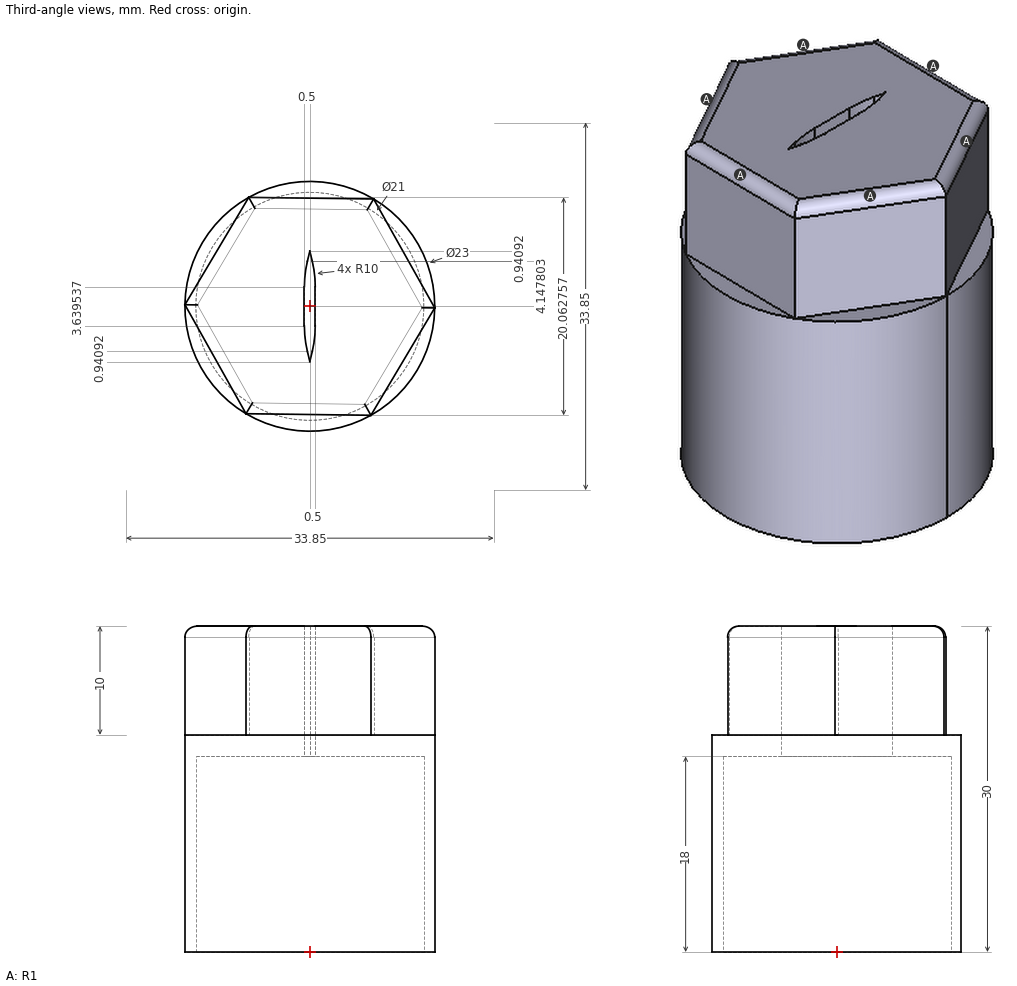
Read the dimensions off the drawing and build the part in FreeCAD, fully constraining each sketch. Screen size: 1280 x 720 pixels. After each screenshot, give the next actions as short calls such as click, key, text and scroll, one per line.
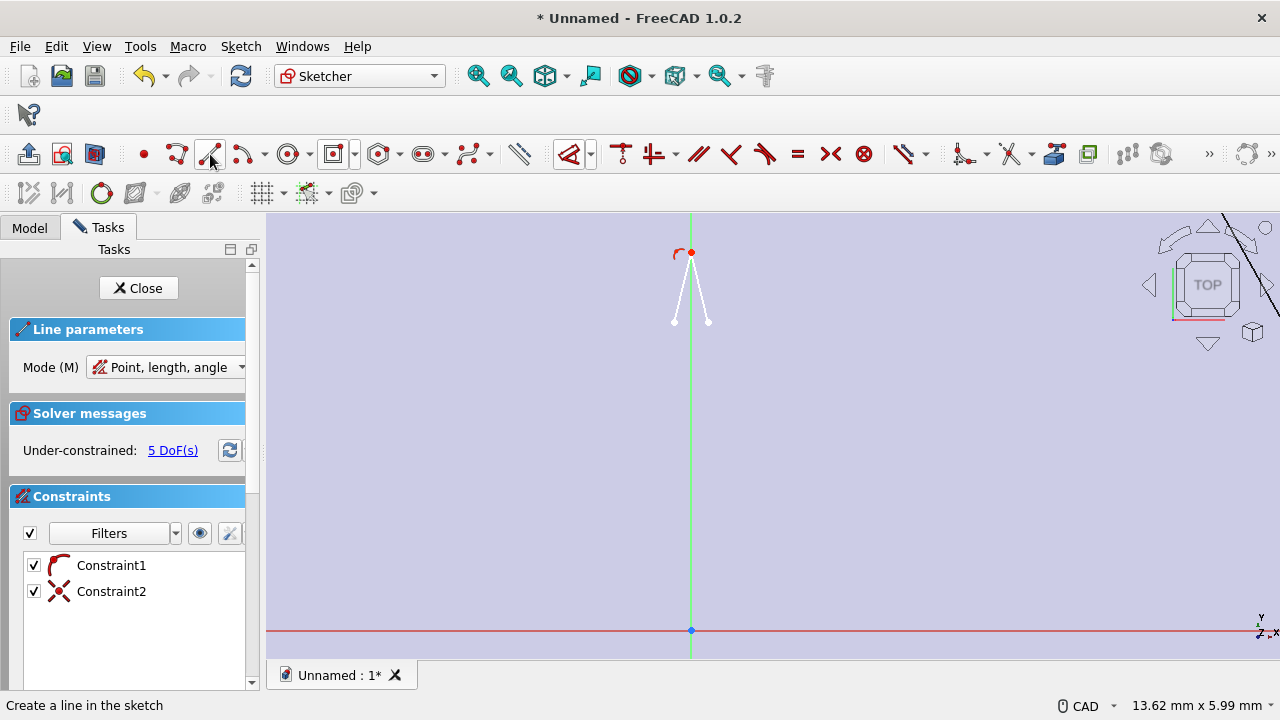
click(654, 495)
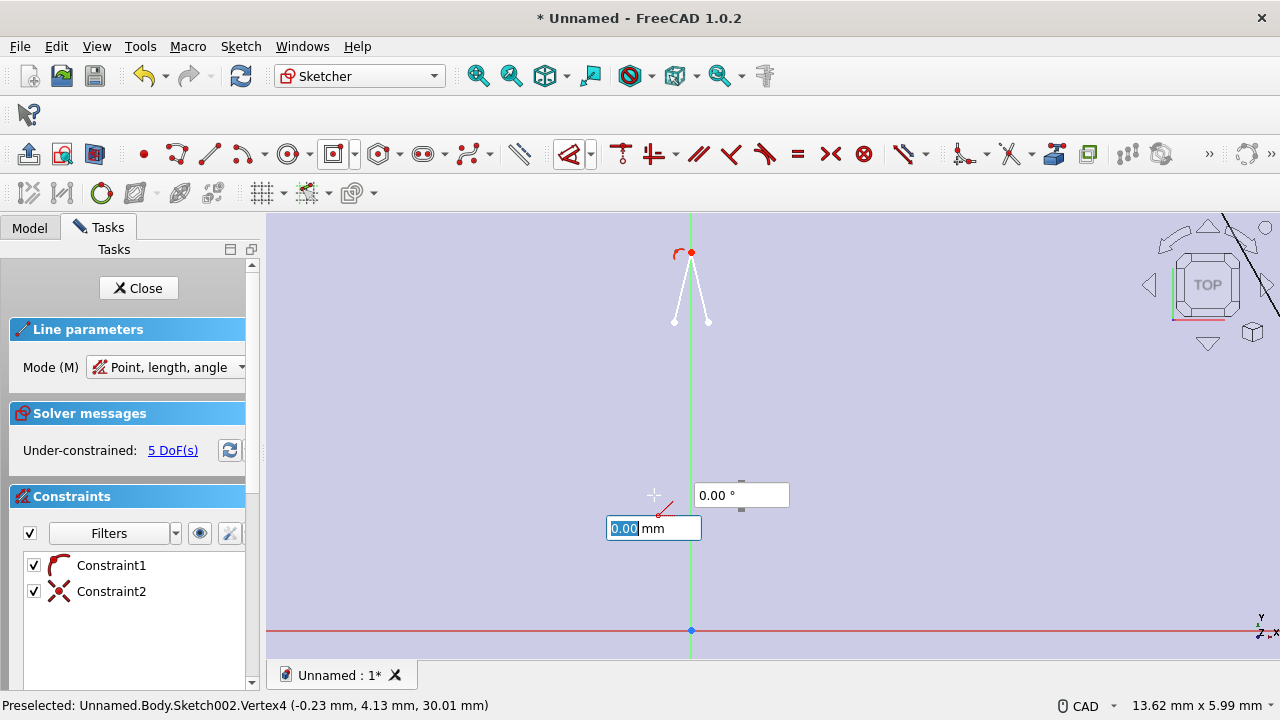
scroll(712, 323, down, 5)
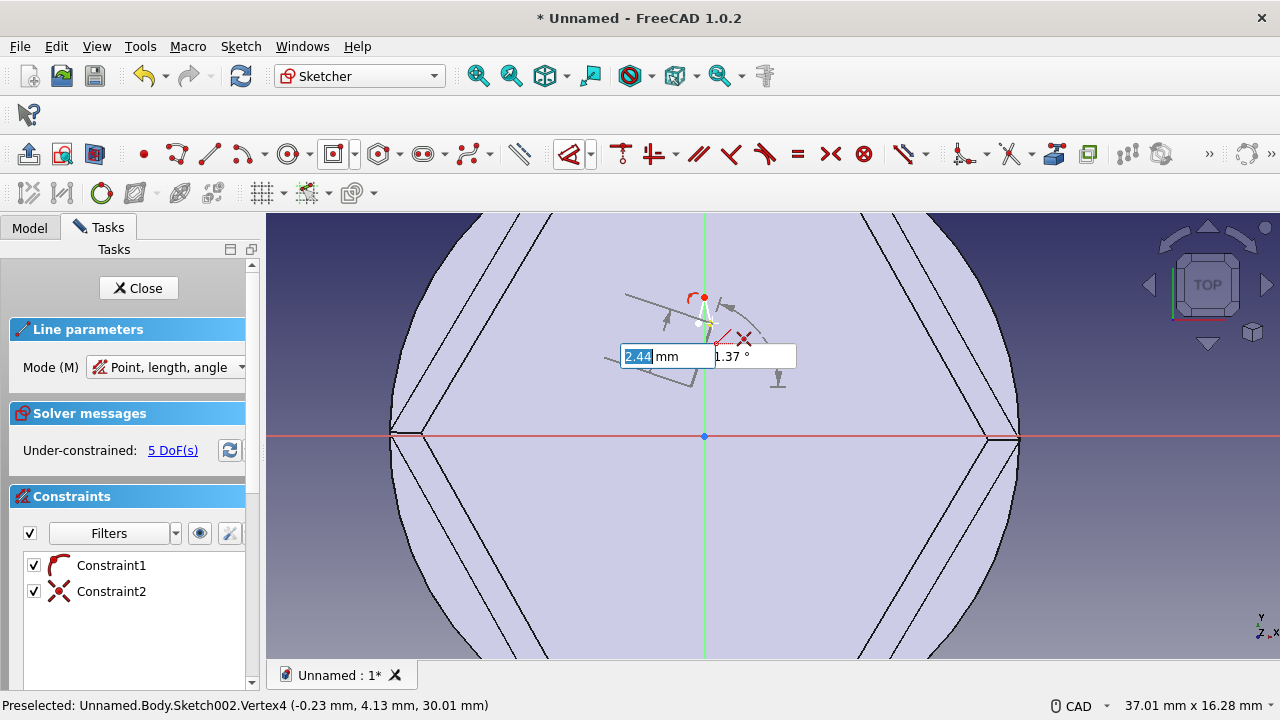
click(691, 486)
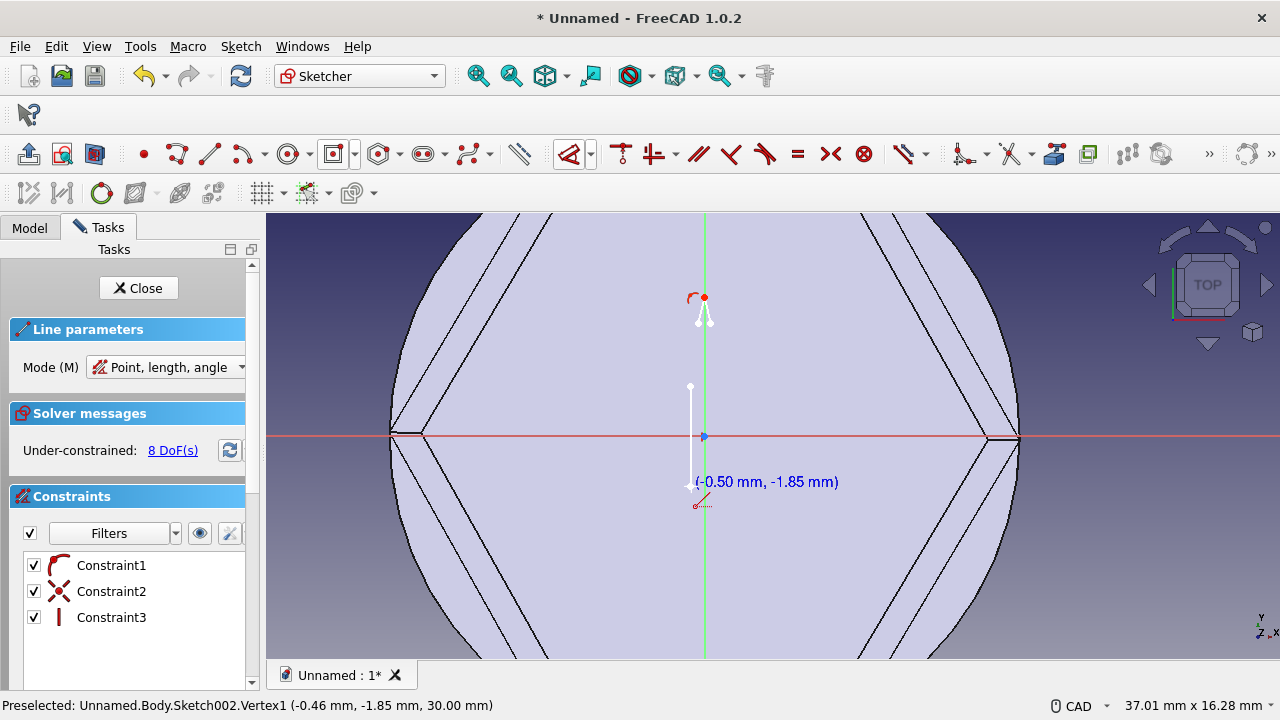
click(177, 154)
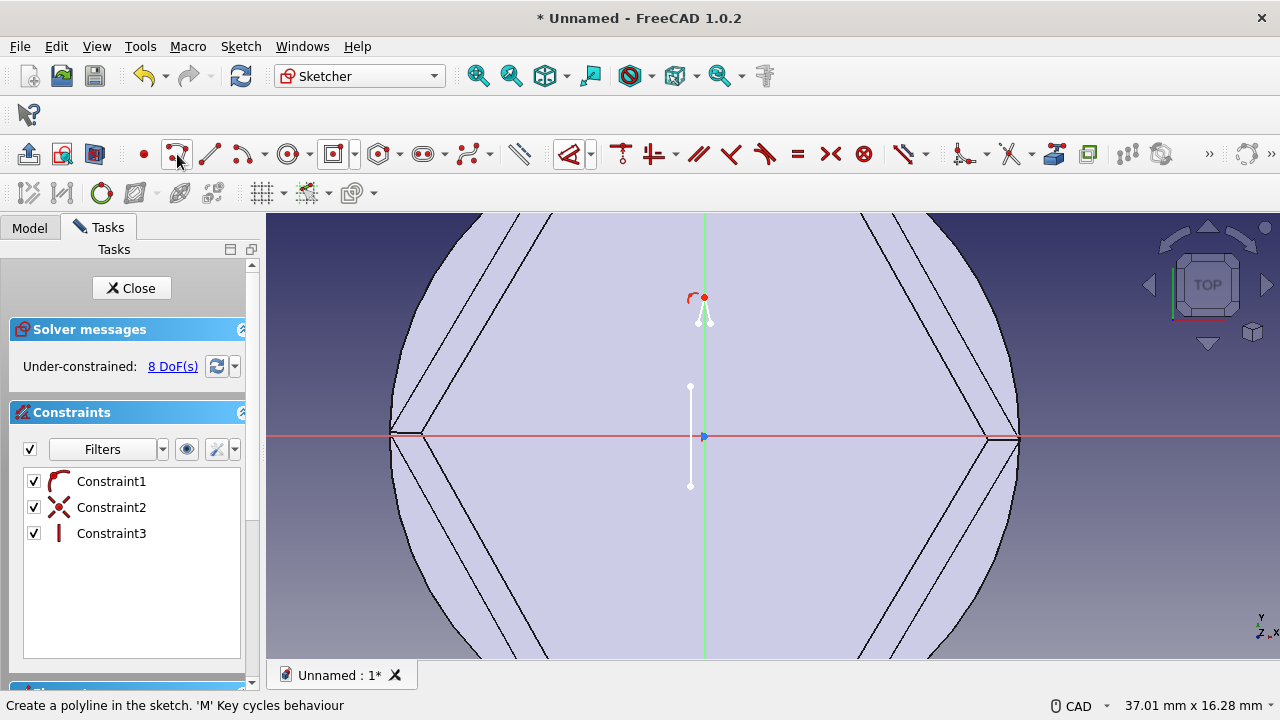
scroll(698, 550, up, 5)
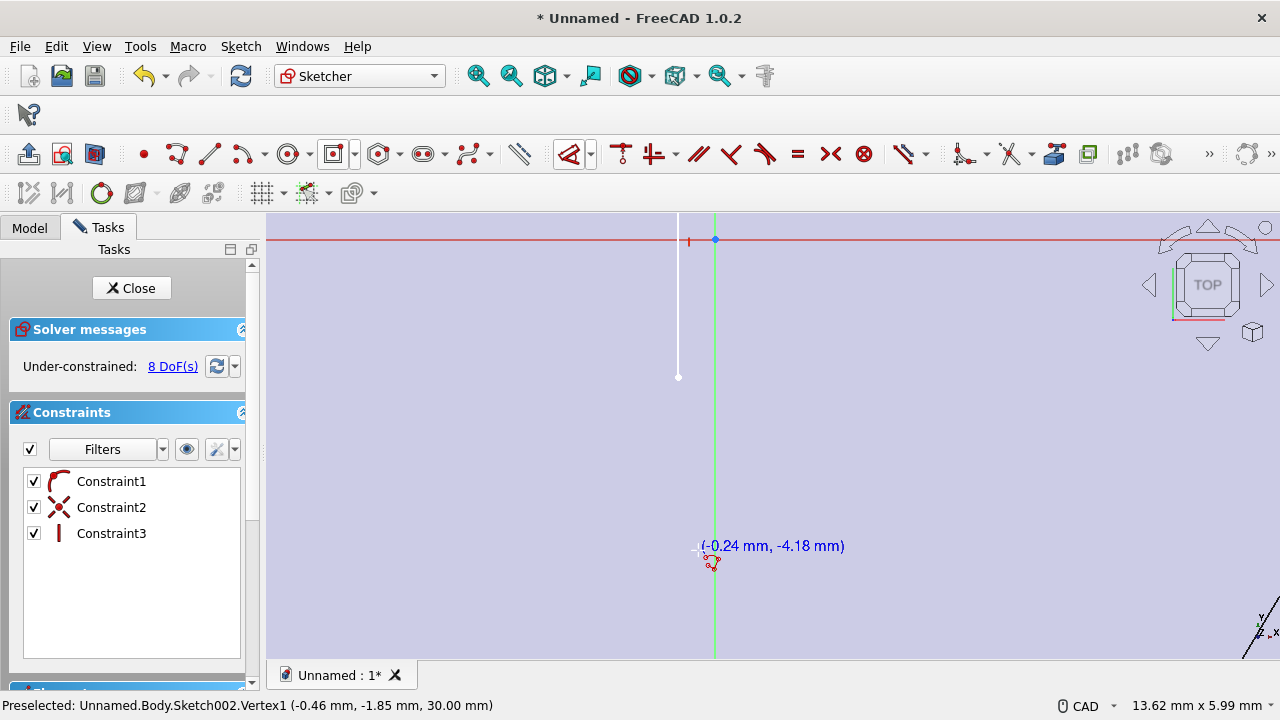
click(698, 549)
click(715, 619)
click(732, 549)
right_click(732, 549)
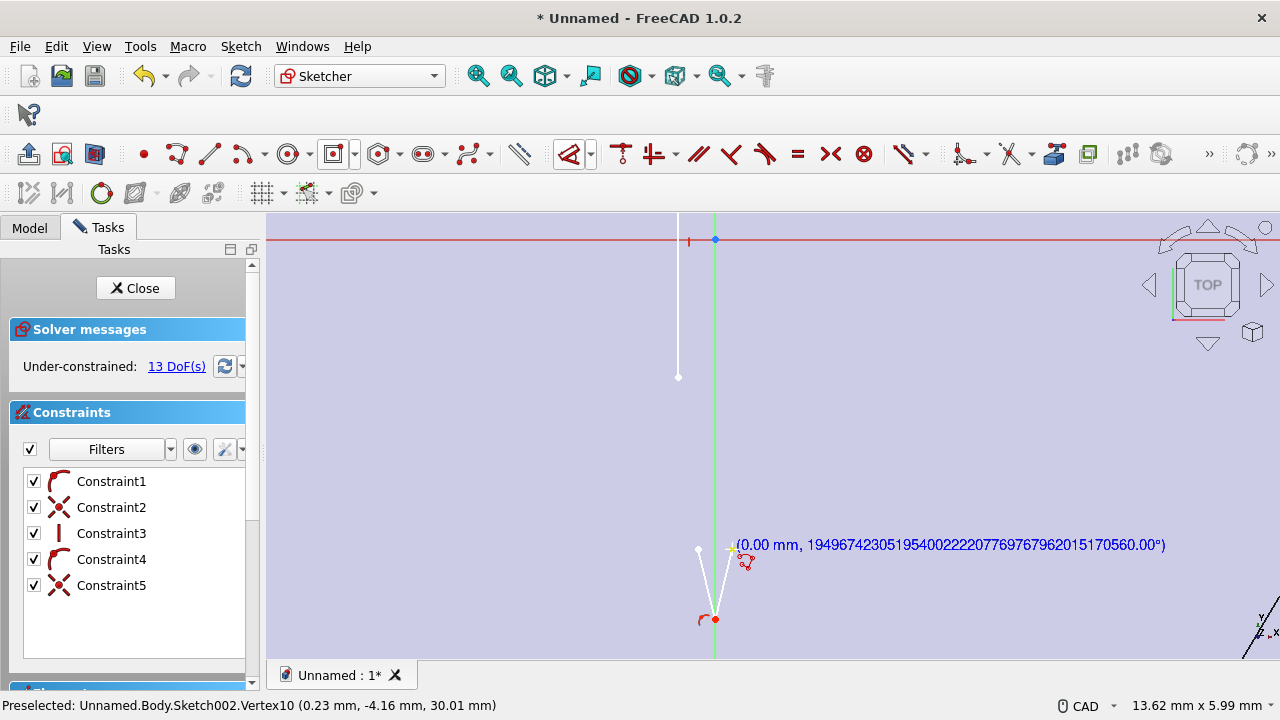
click(210, 154)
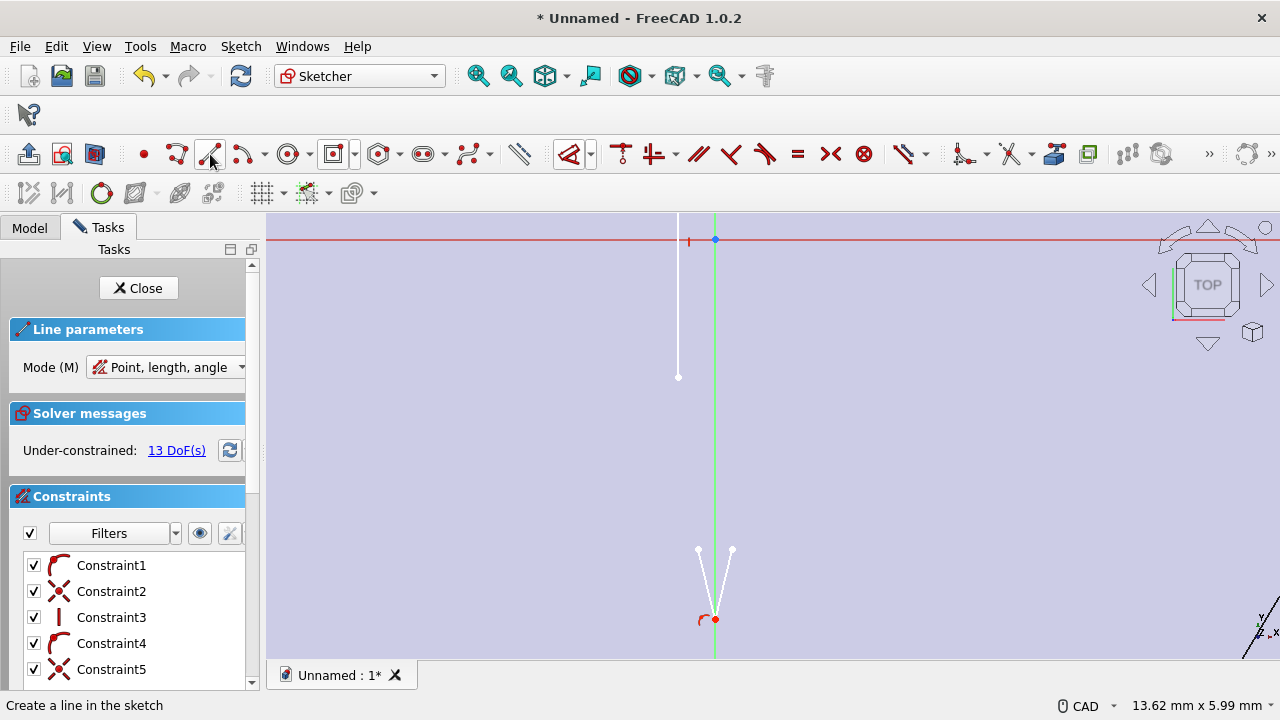
click(752, 375)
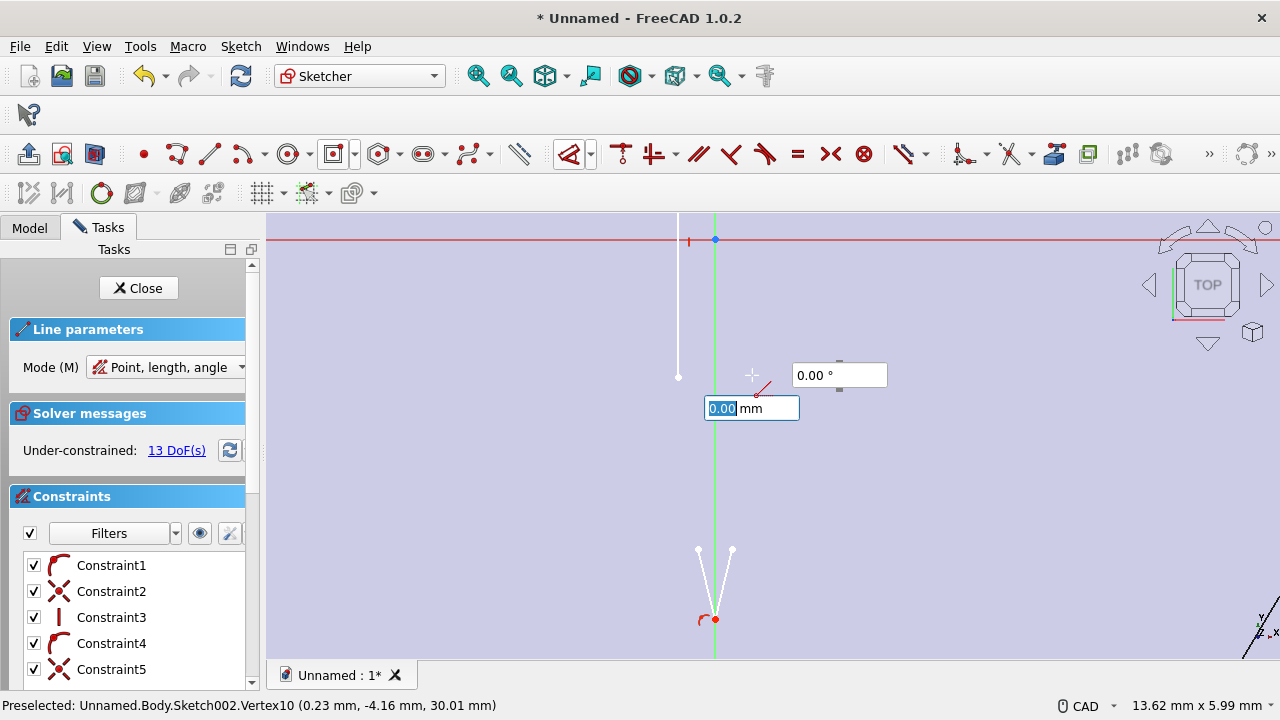
scroll(698, 550, down, 5)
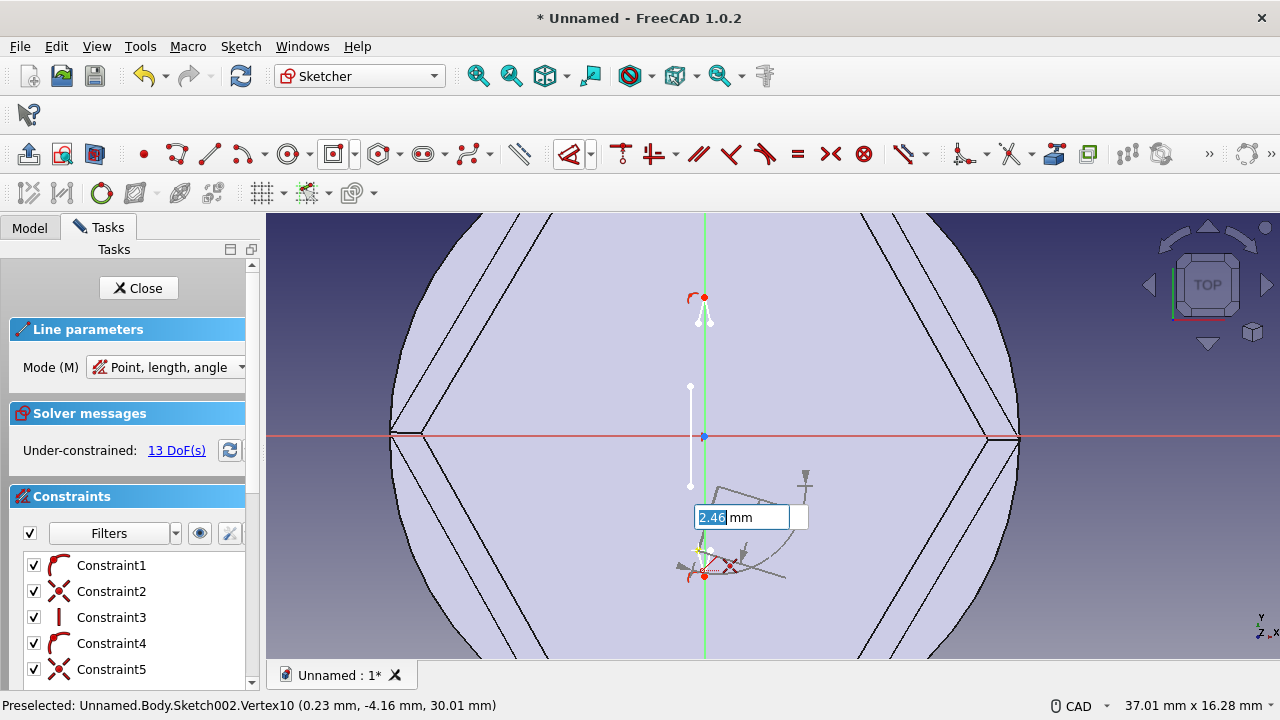
click(718, 387)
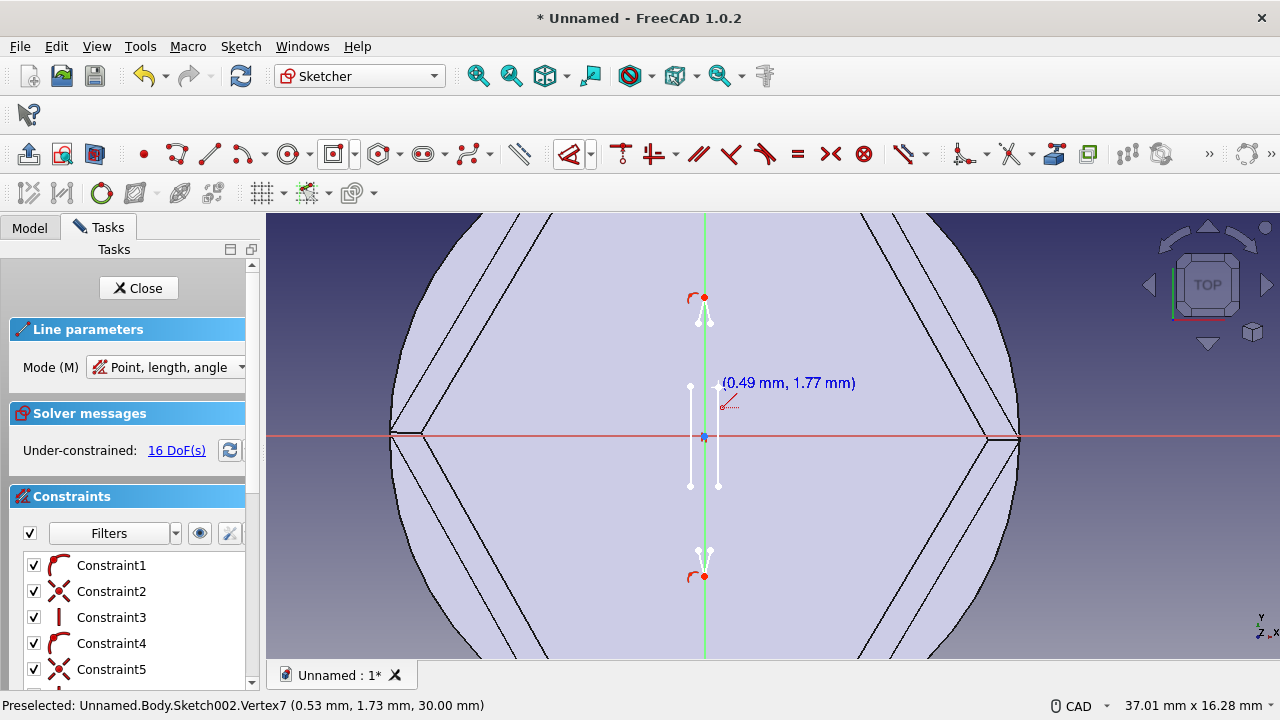
key(g)
key(3)
key(a)